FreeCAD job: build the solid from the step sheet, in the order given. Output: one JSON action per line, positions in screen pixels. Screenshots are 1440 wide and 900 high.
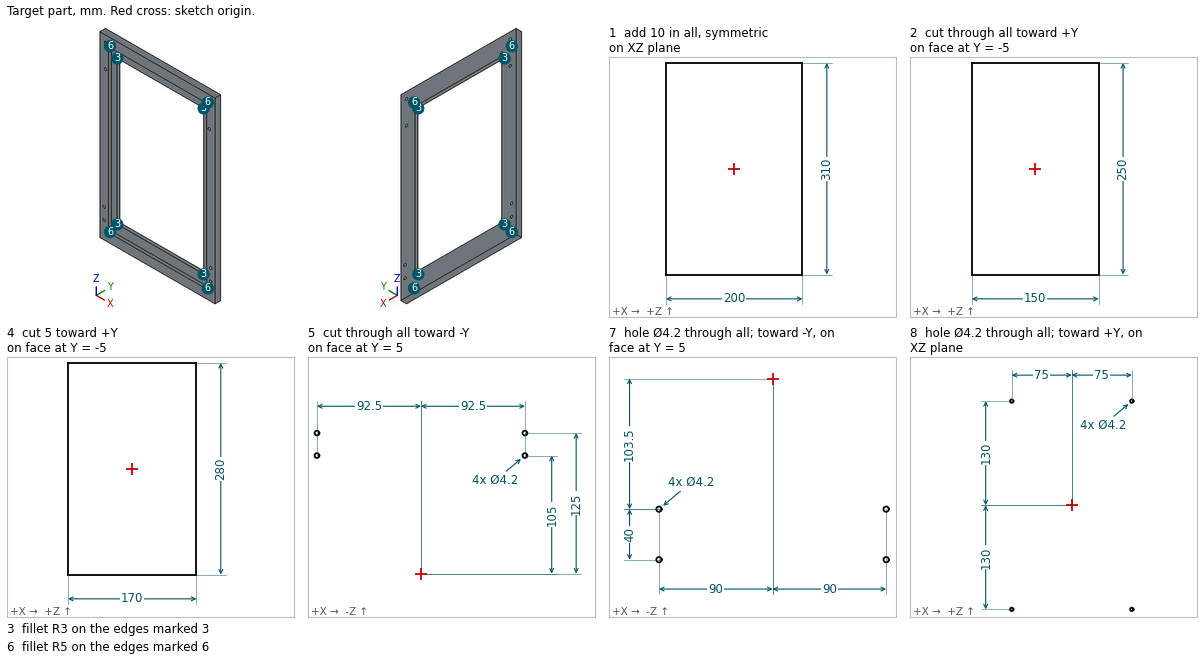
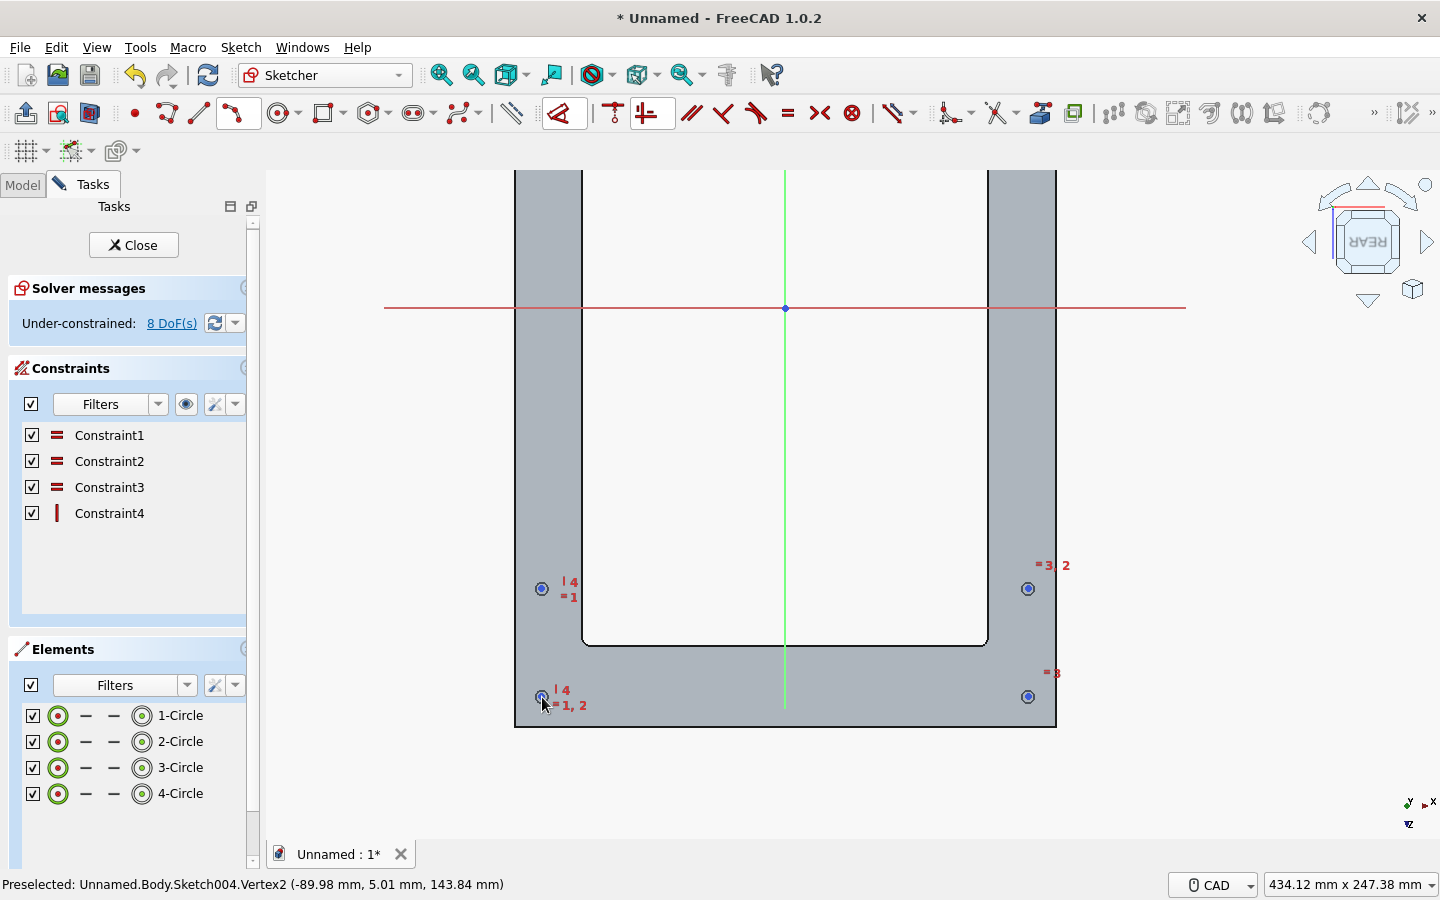
{"action": "left_click", "coordinate": [542, 589]}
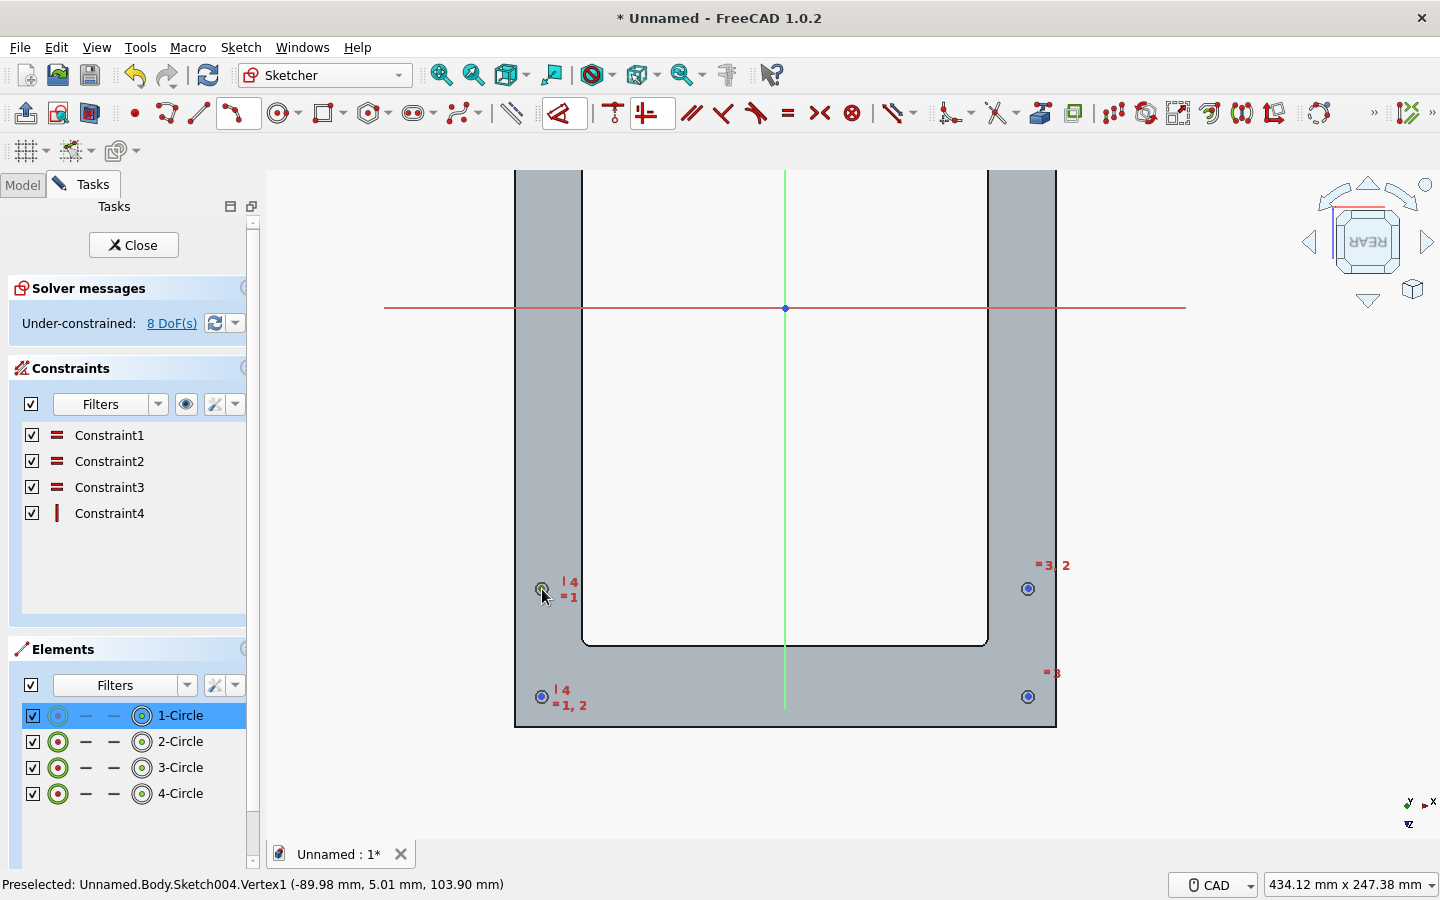
{"action": "left_click", "coordinate": [1028, 589]}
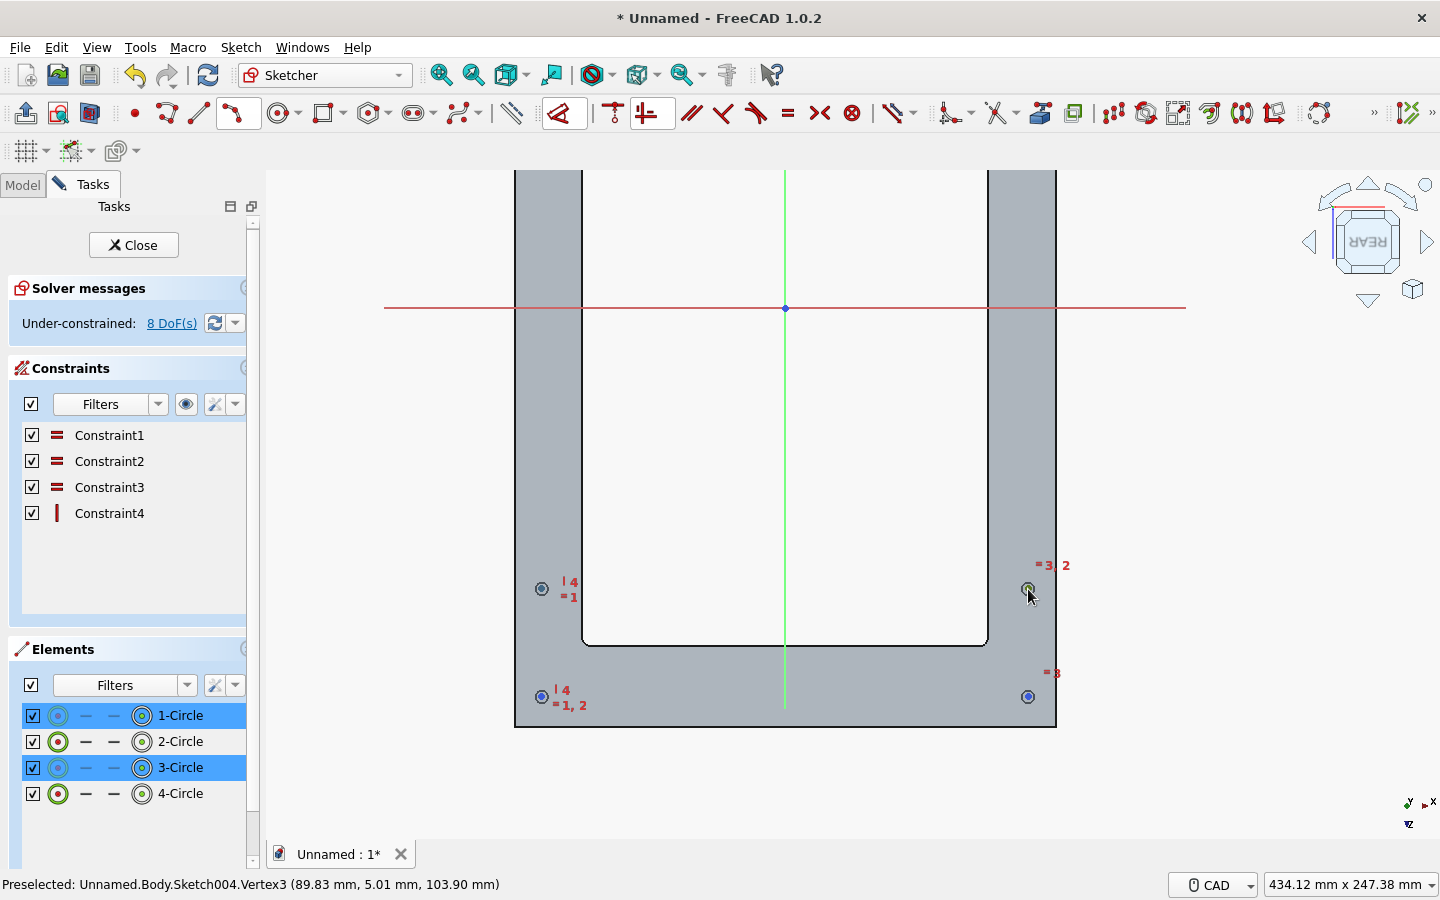
{"action": "key", "text": "h"}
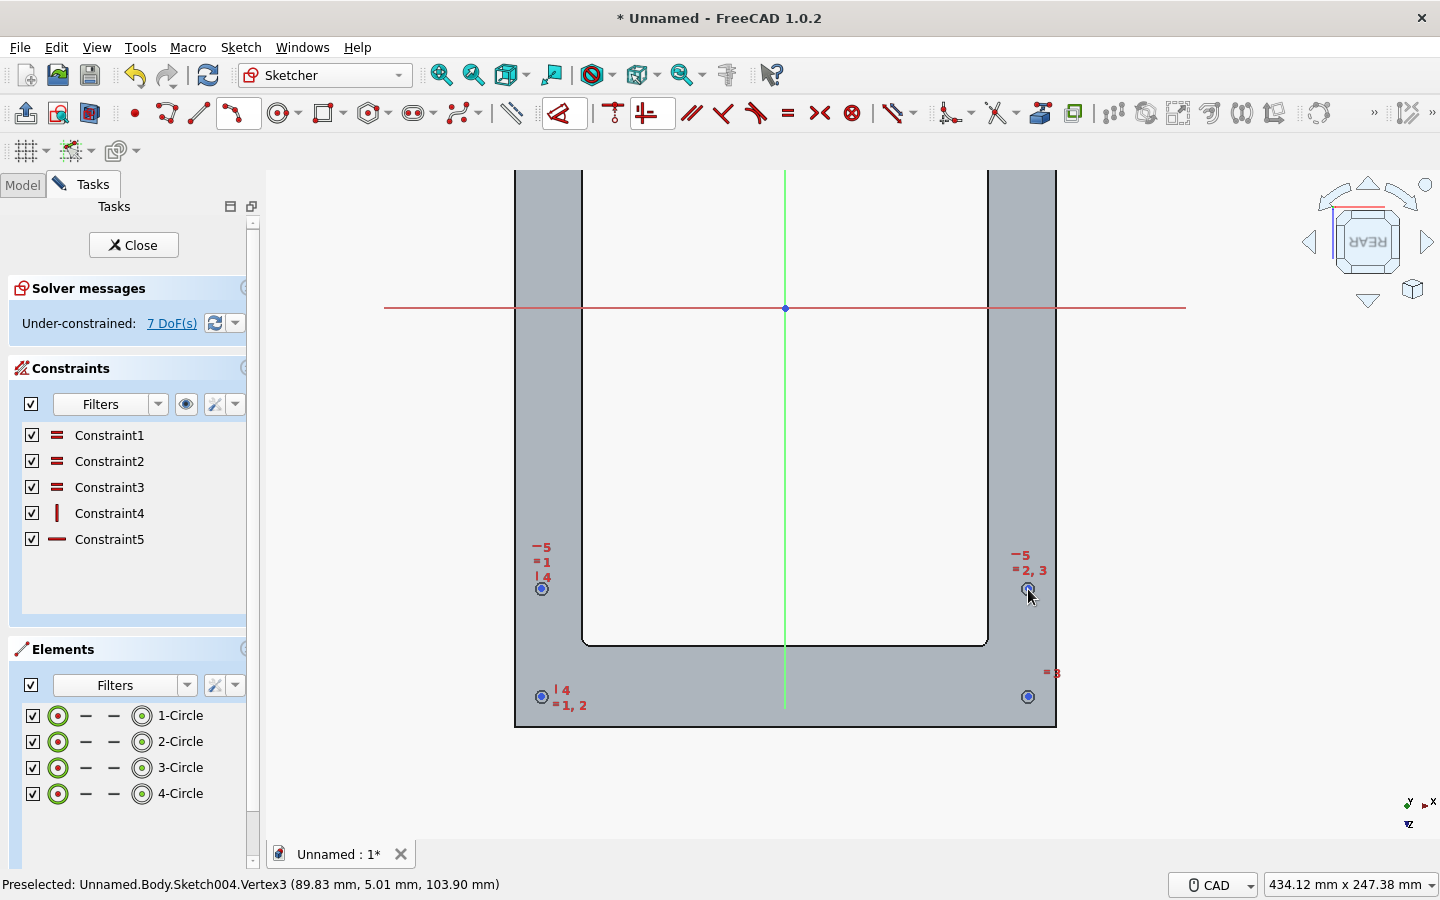
{"action": "left_click", "coordinate": [1028, 589]}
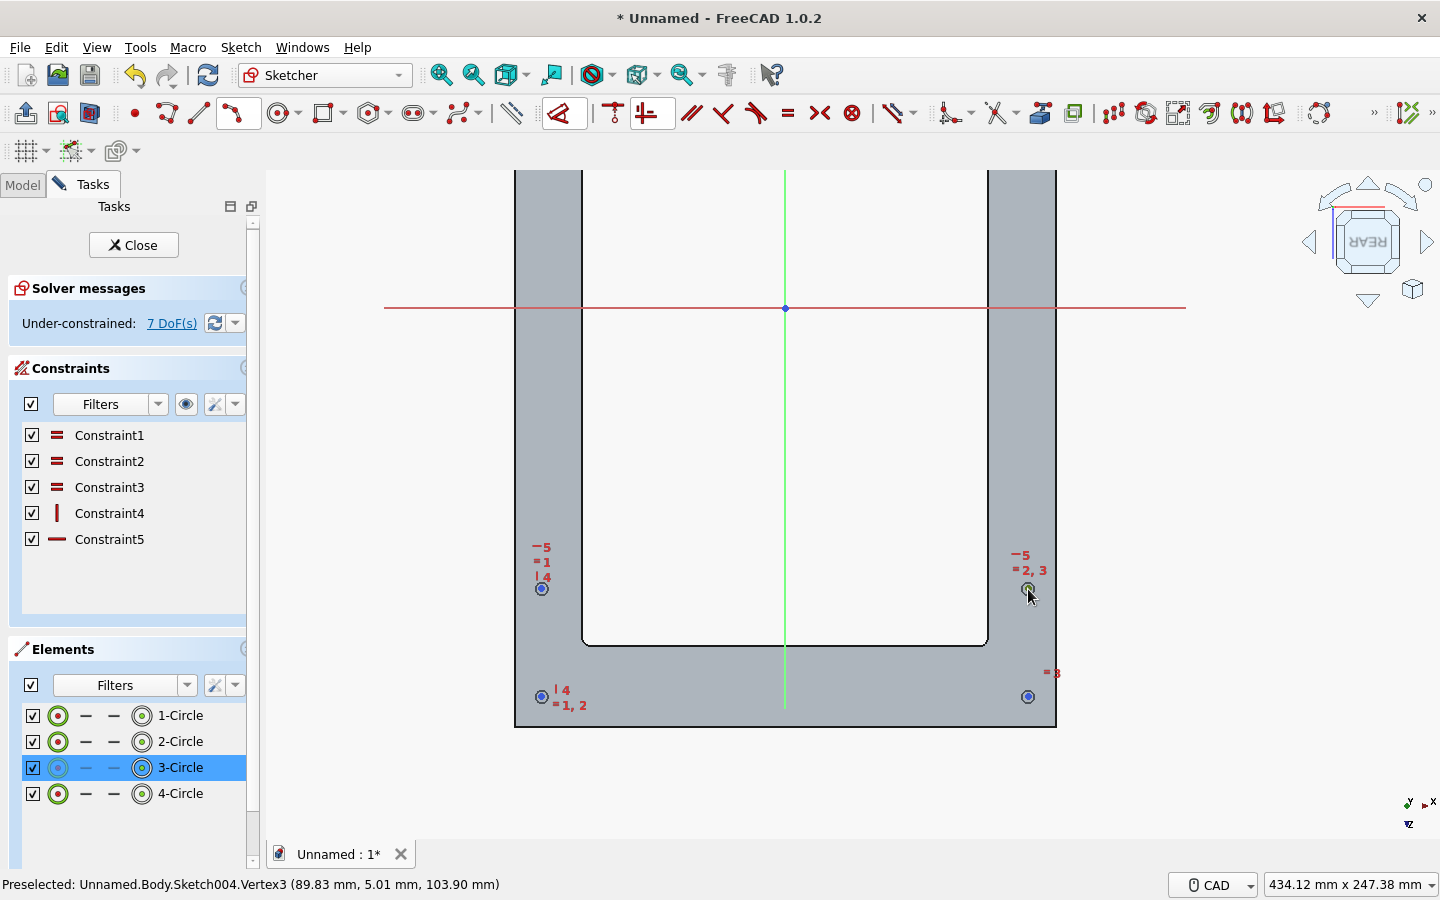
{"action": "left_click", "coordinate": [1028, 697]}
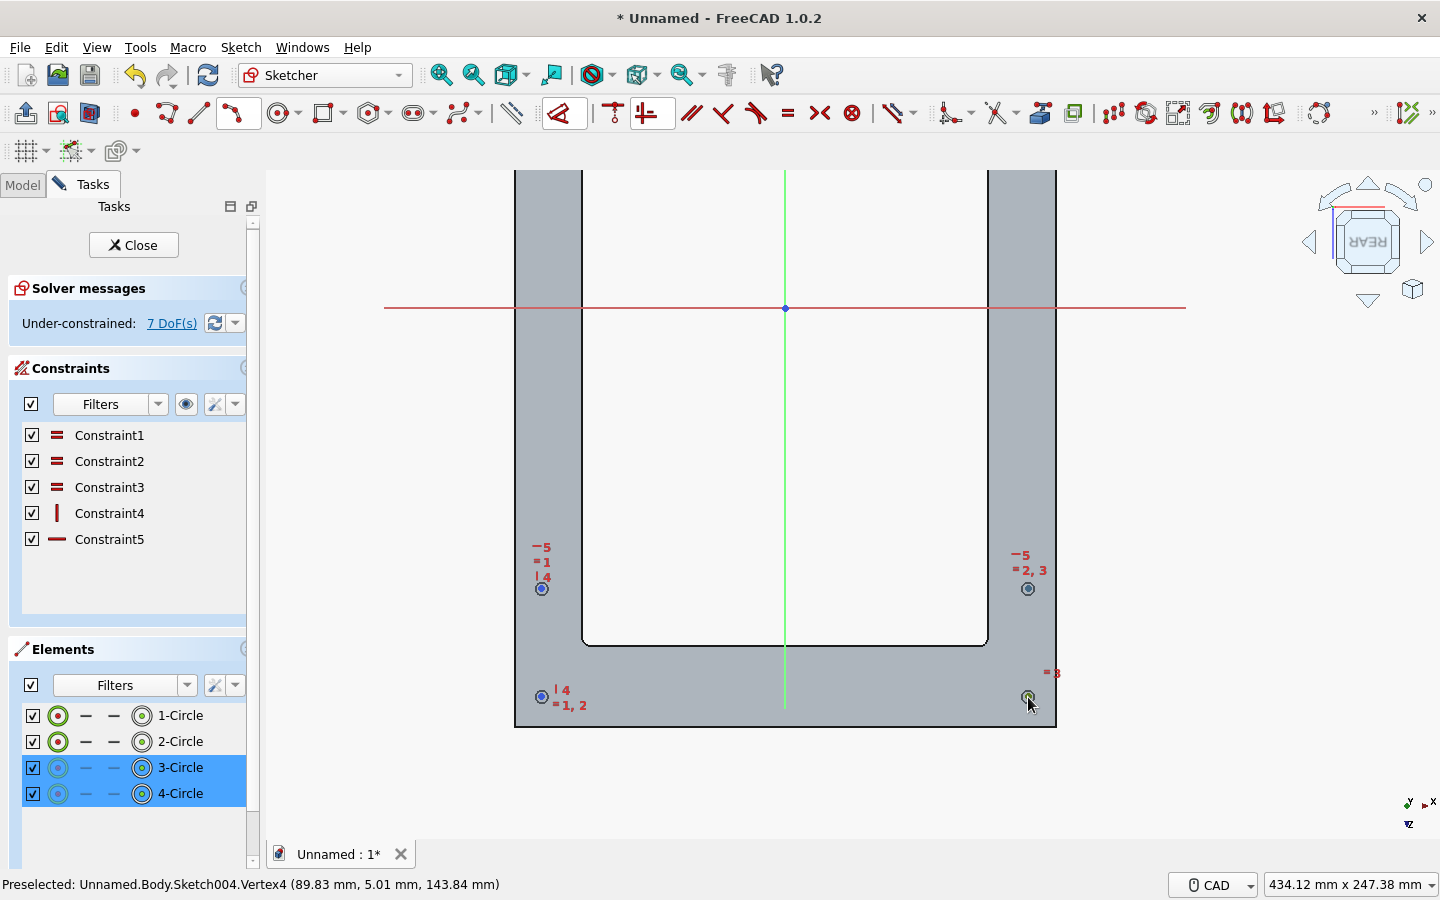
{"action": "key", "text": "v"}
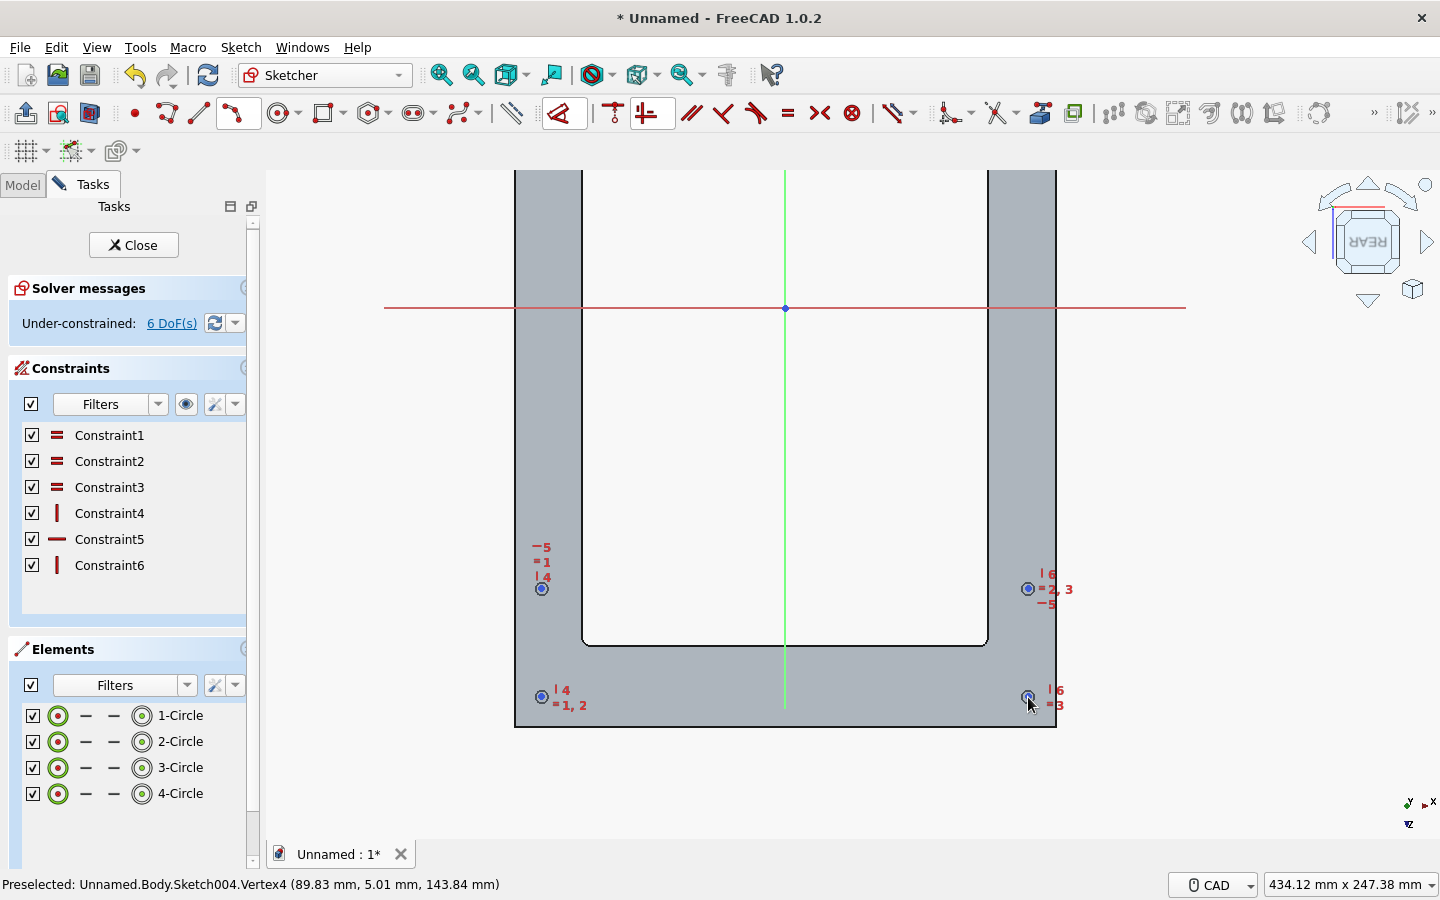
{"action": "left_click", "coordinate": [542, 697]}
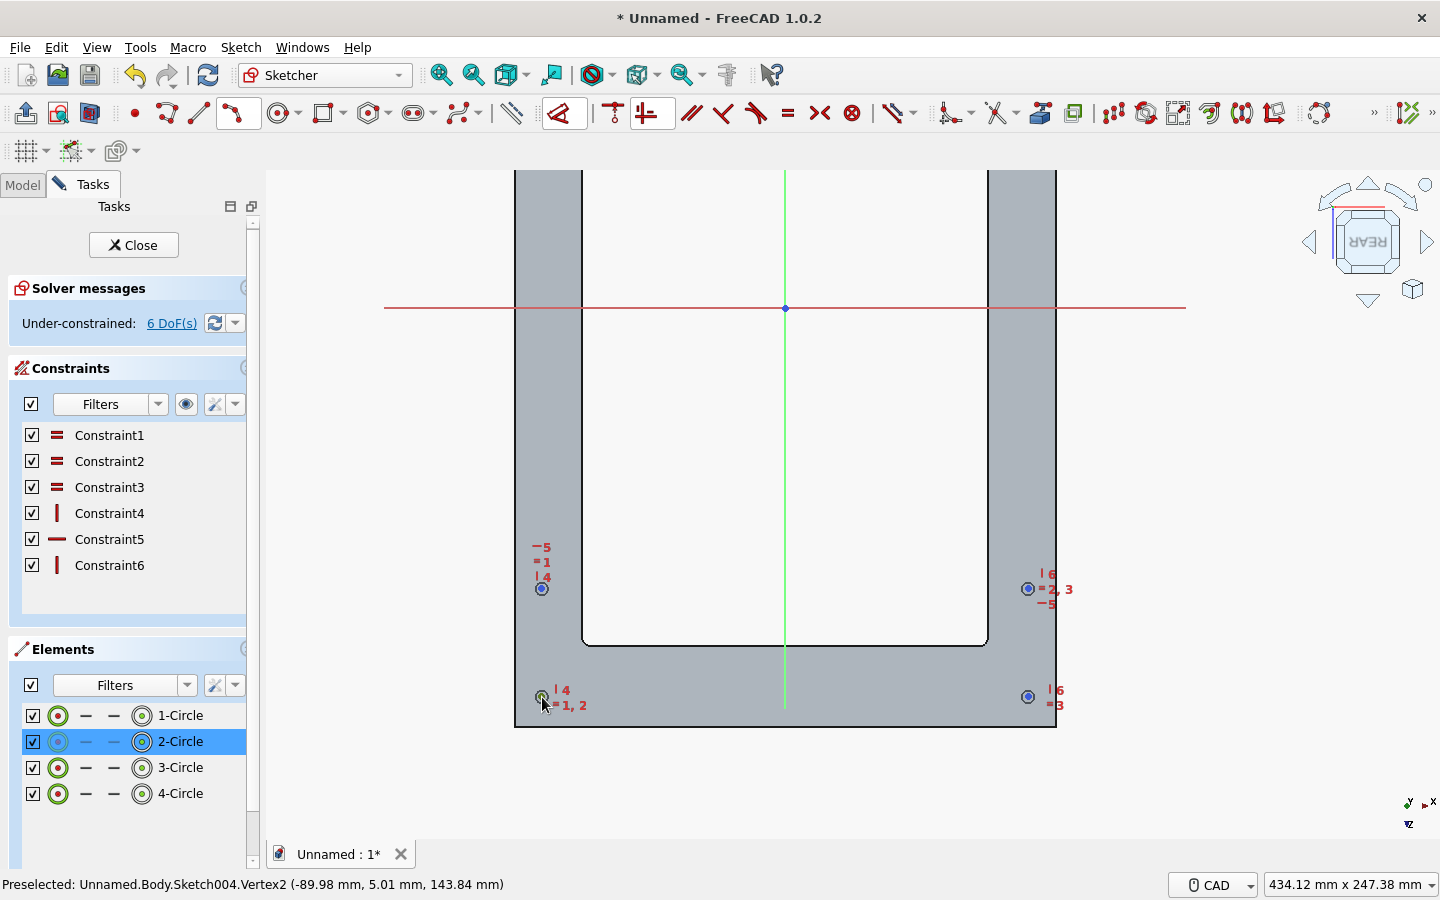
{"action": "left_click", "coordinate": [1028, 697]}